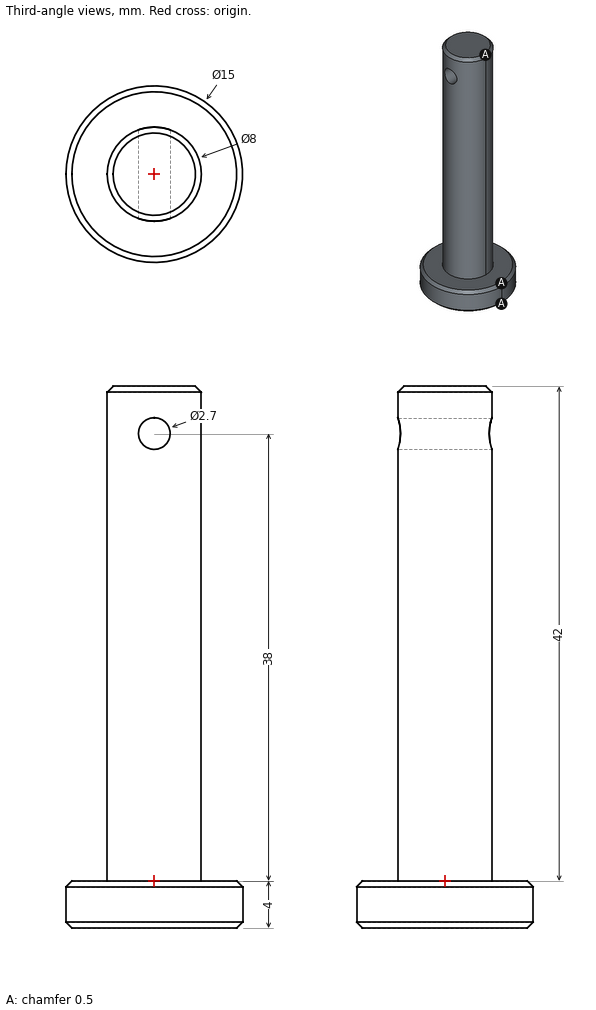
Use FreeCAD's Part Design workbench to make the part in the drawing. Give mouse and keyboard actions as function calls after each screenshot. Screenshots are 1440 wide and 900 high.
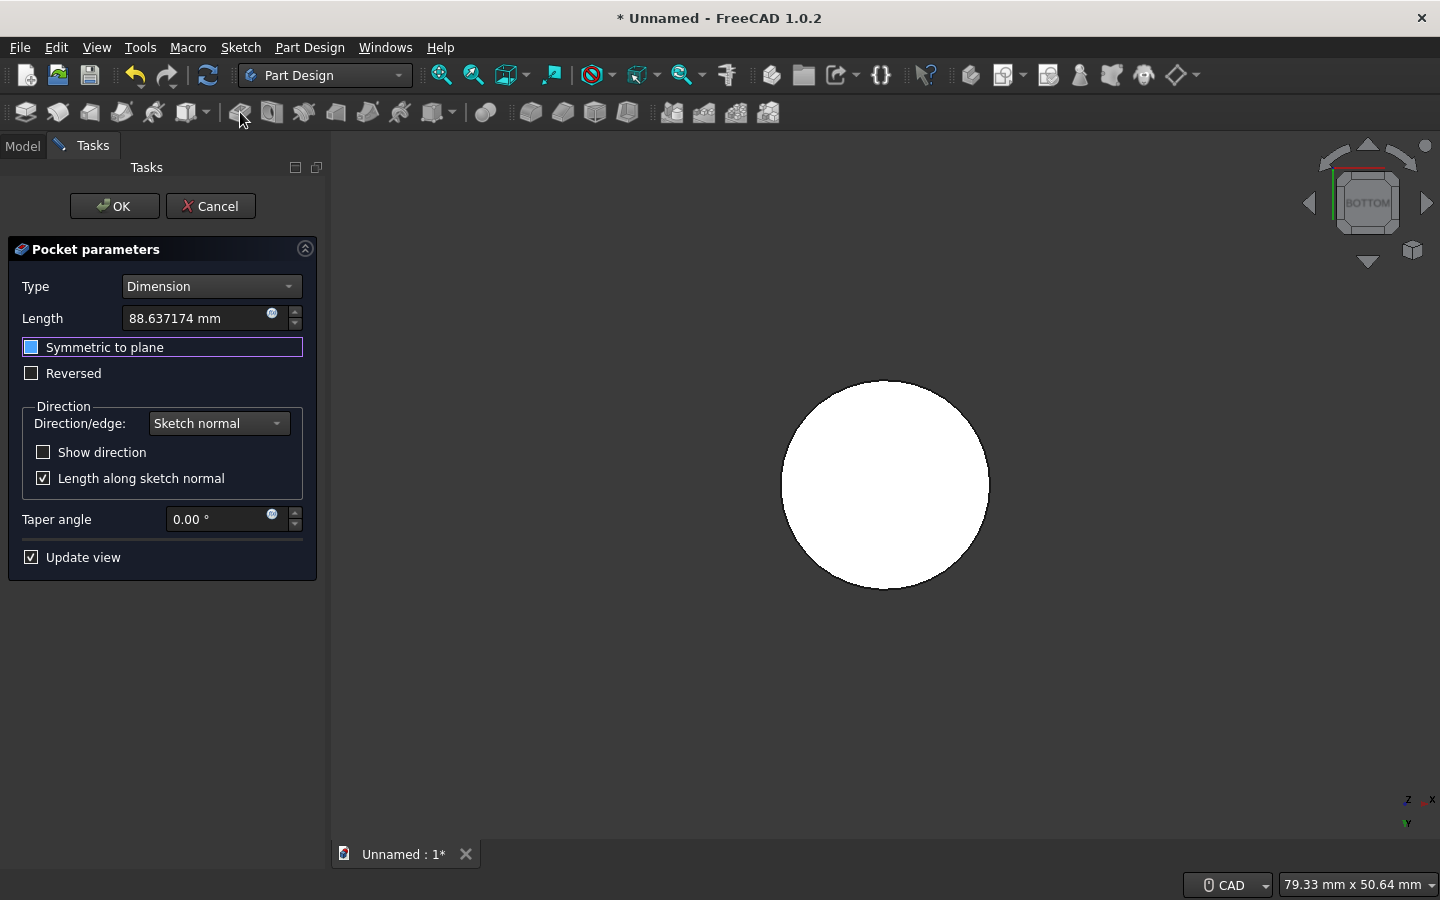
click(30, 347)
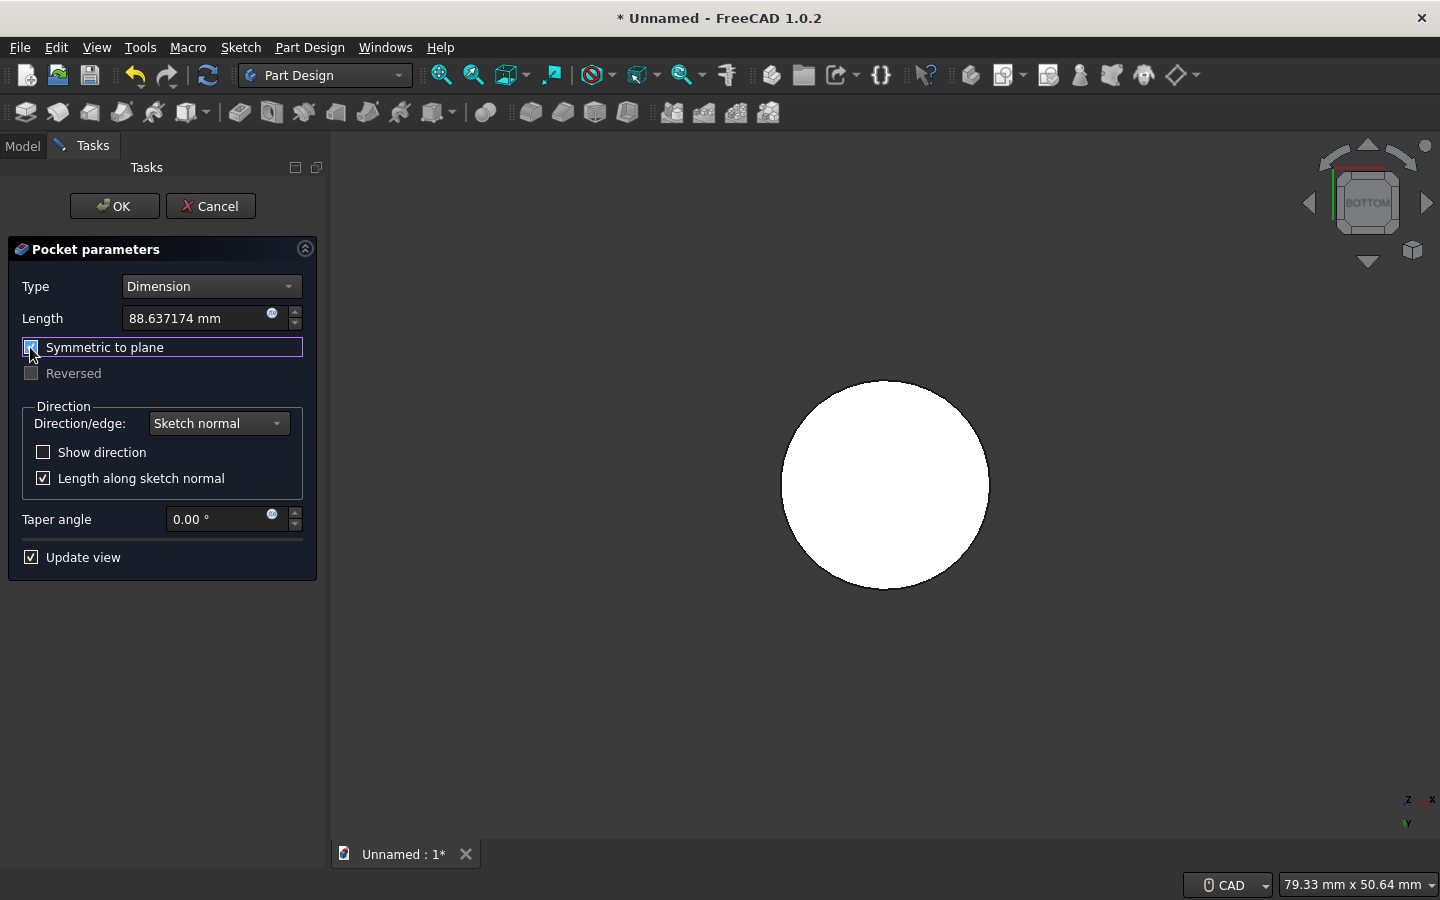
click(115, 206)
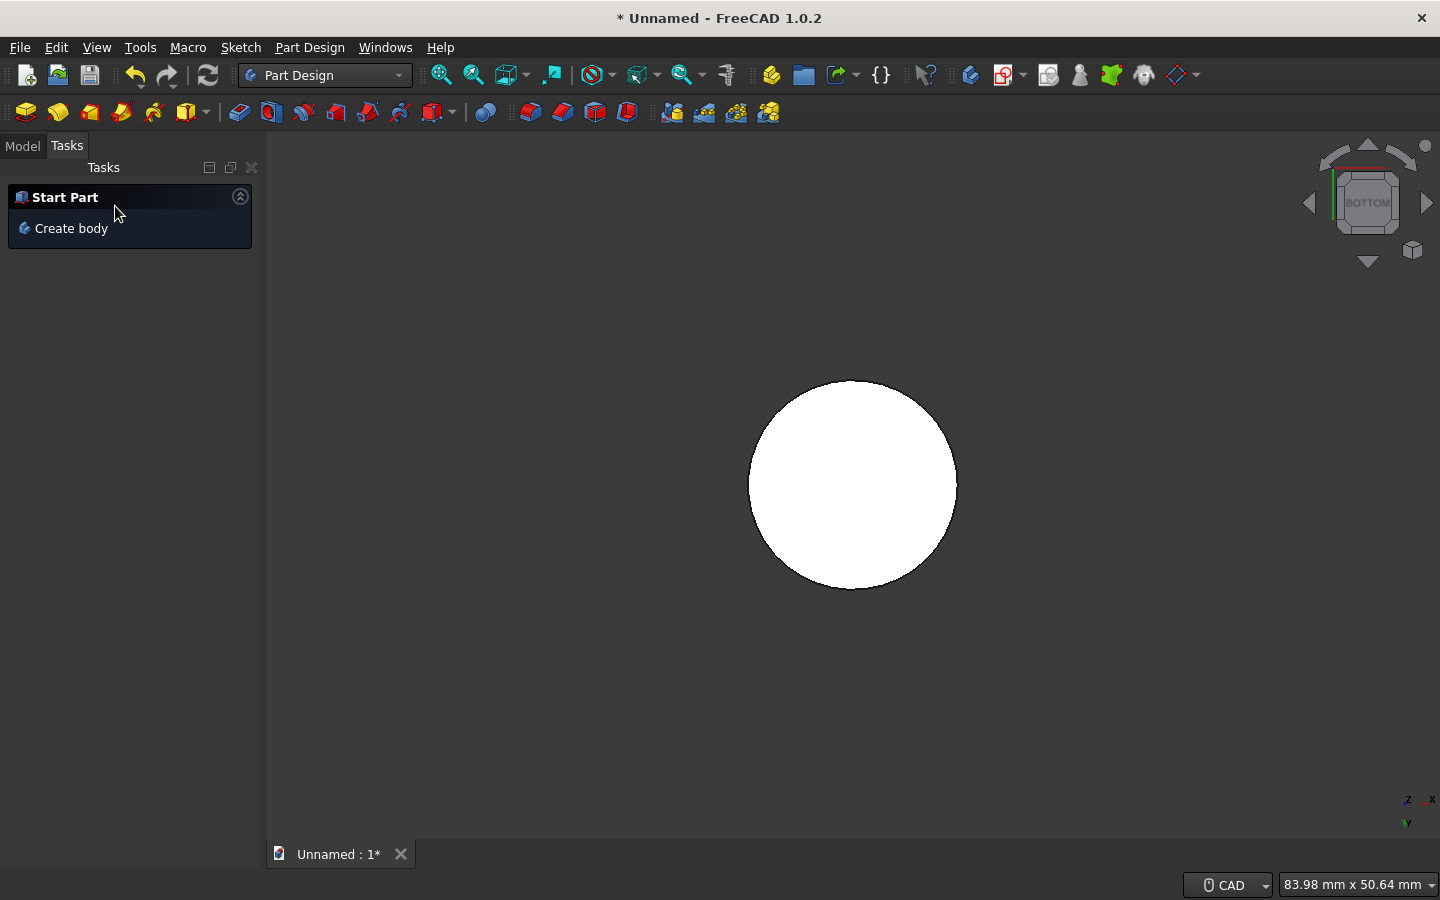
key(v)
key(f)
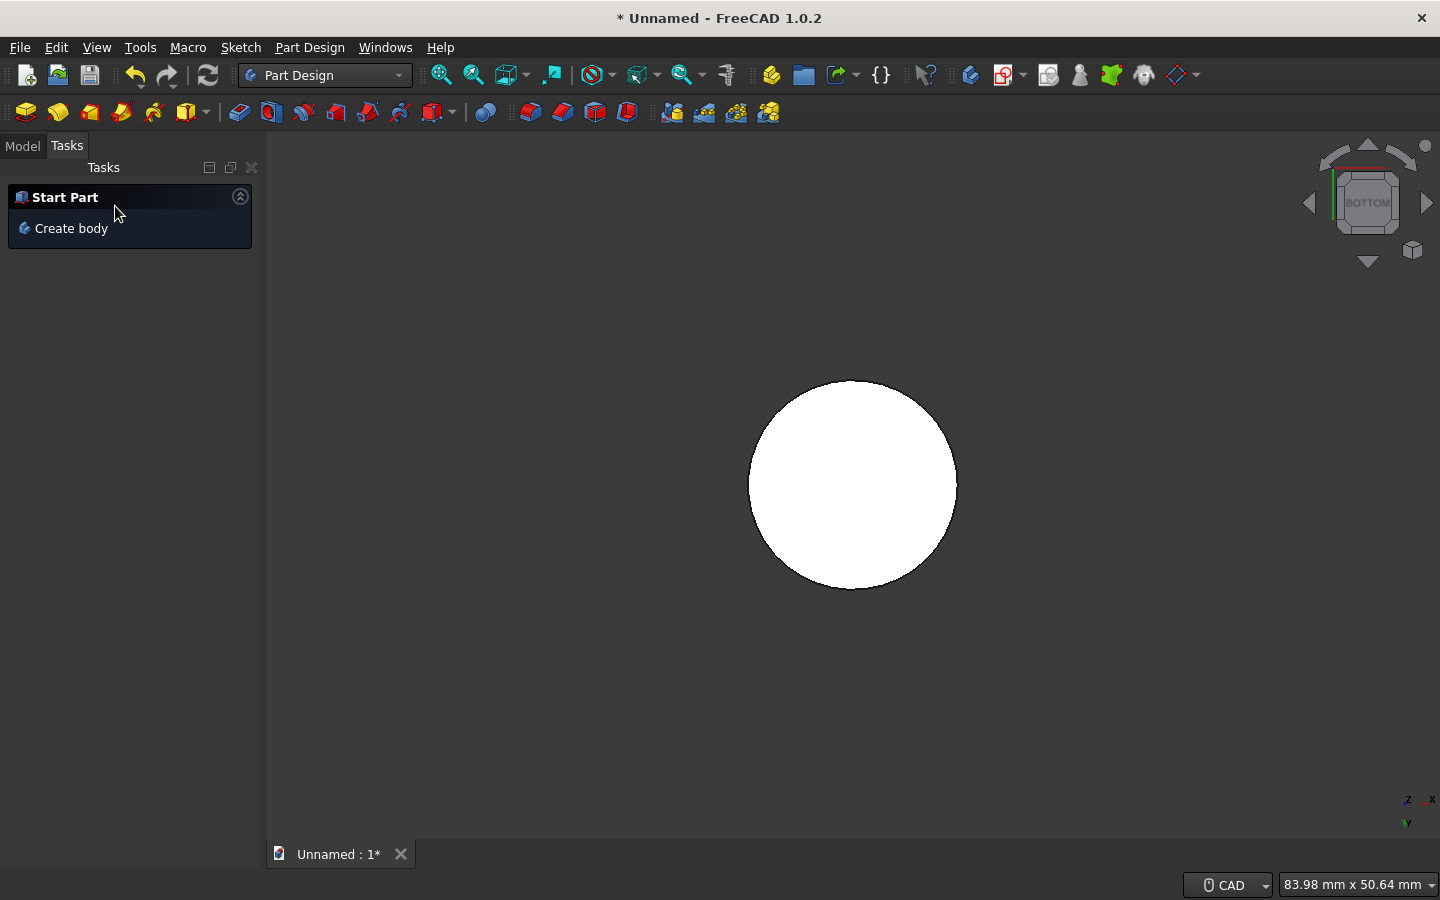
click(748, 484)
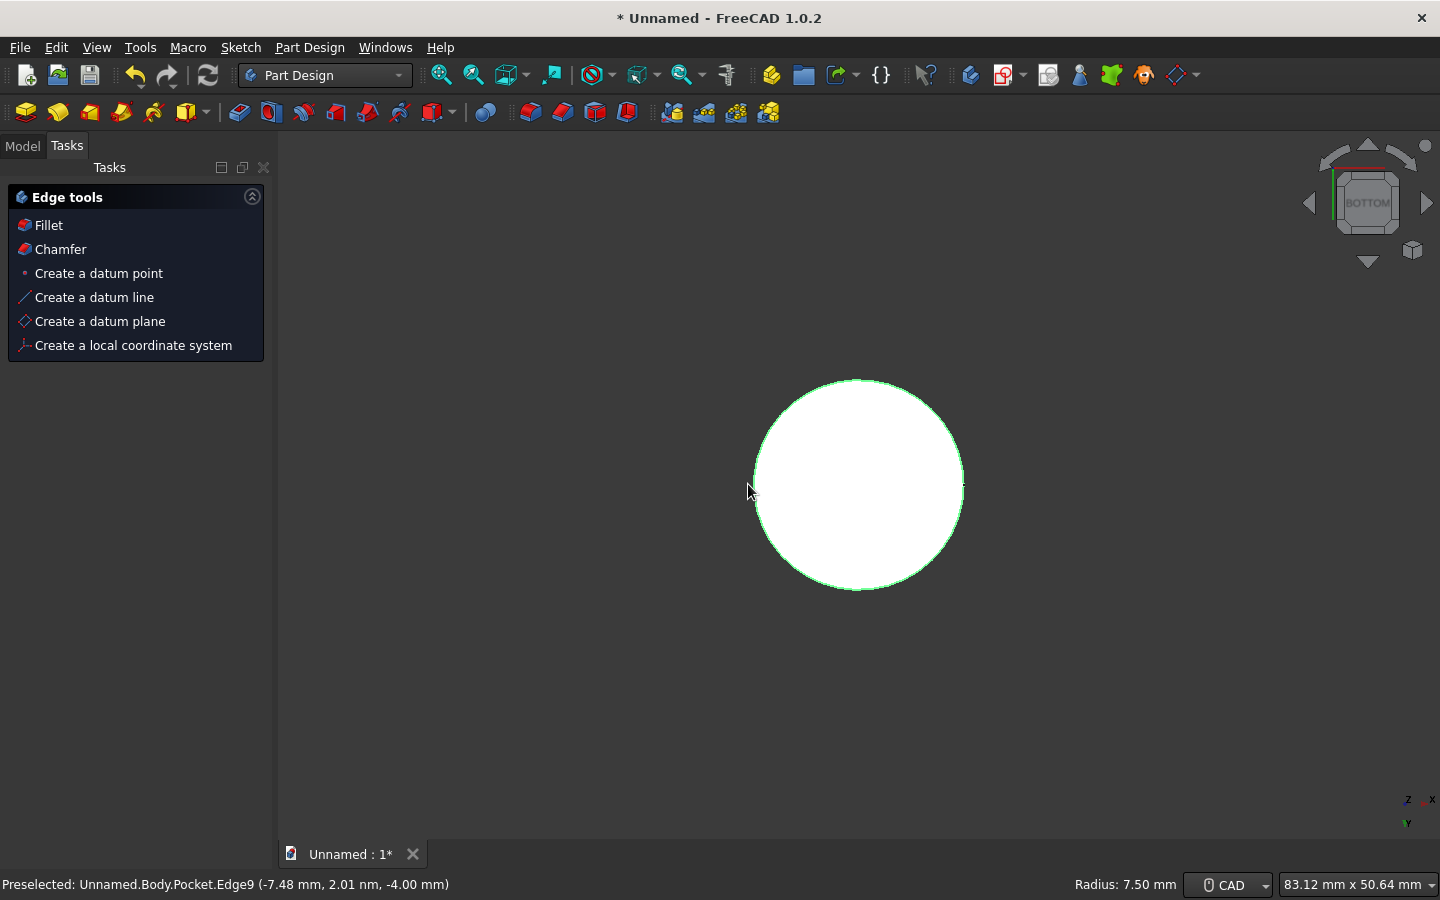
key(0)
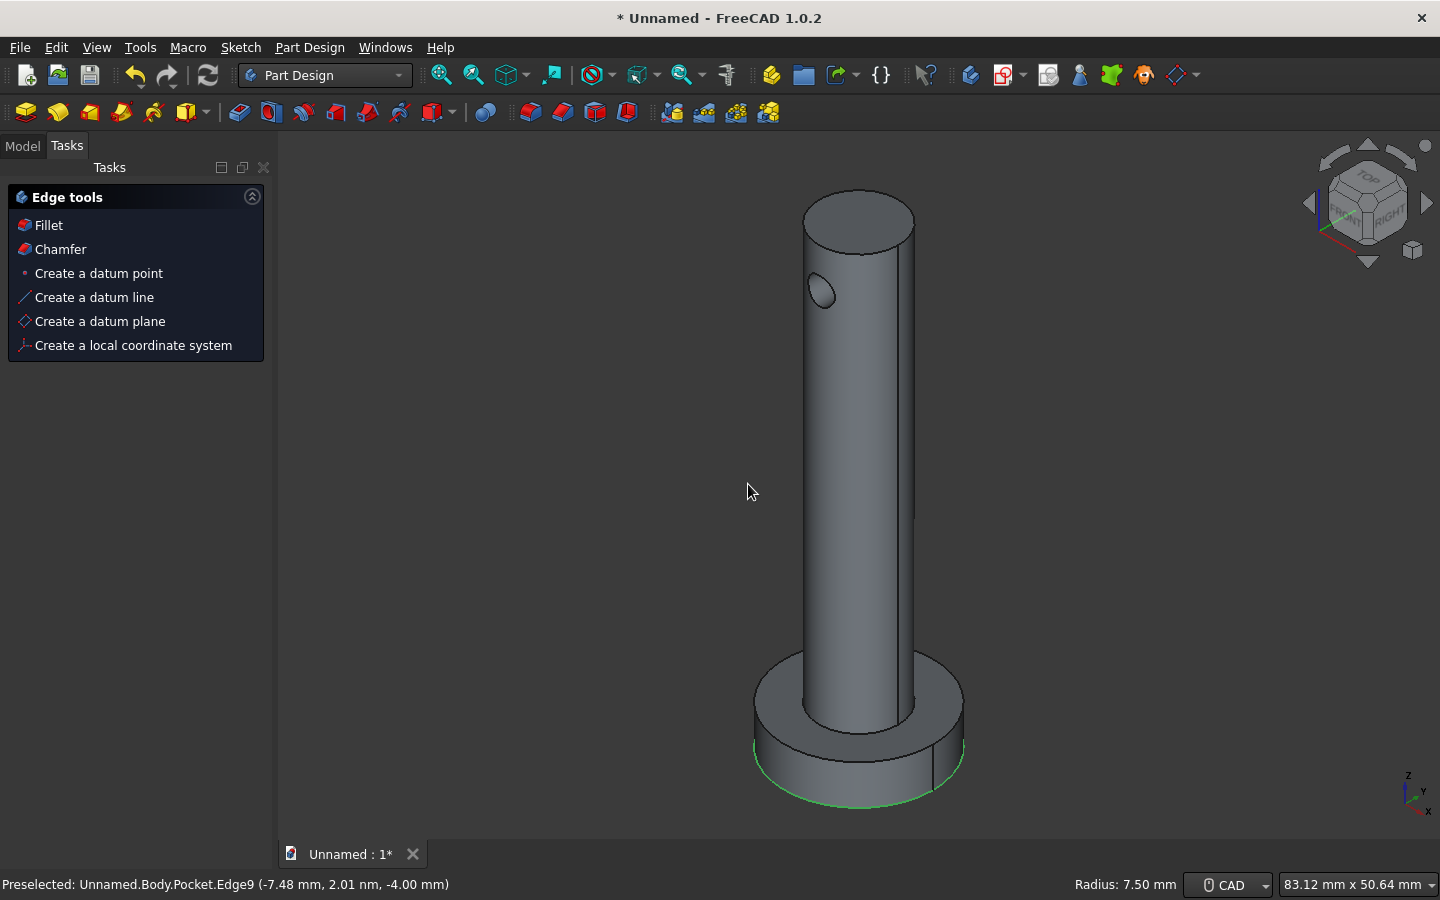
click(809, 236, ctrl)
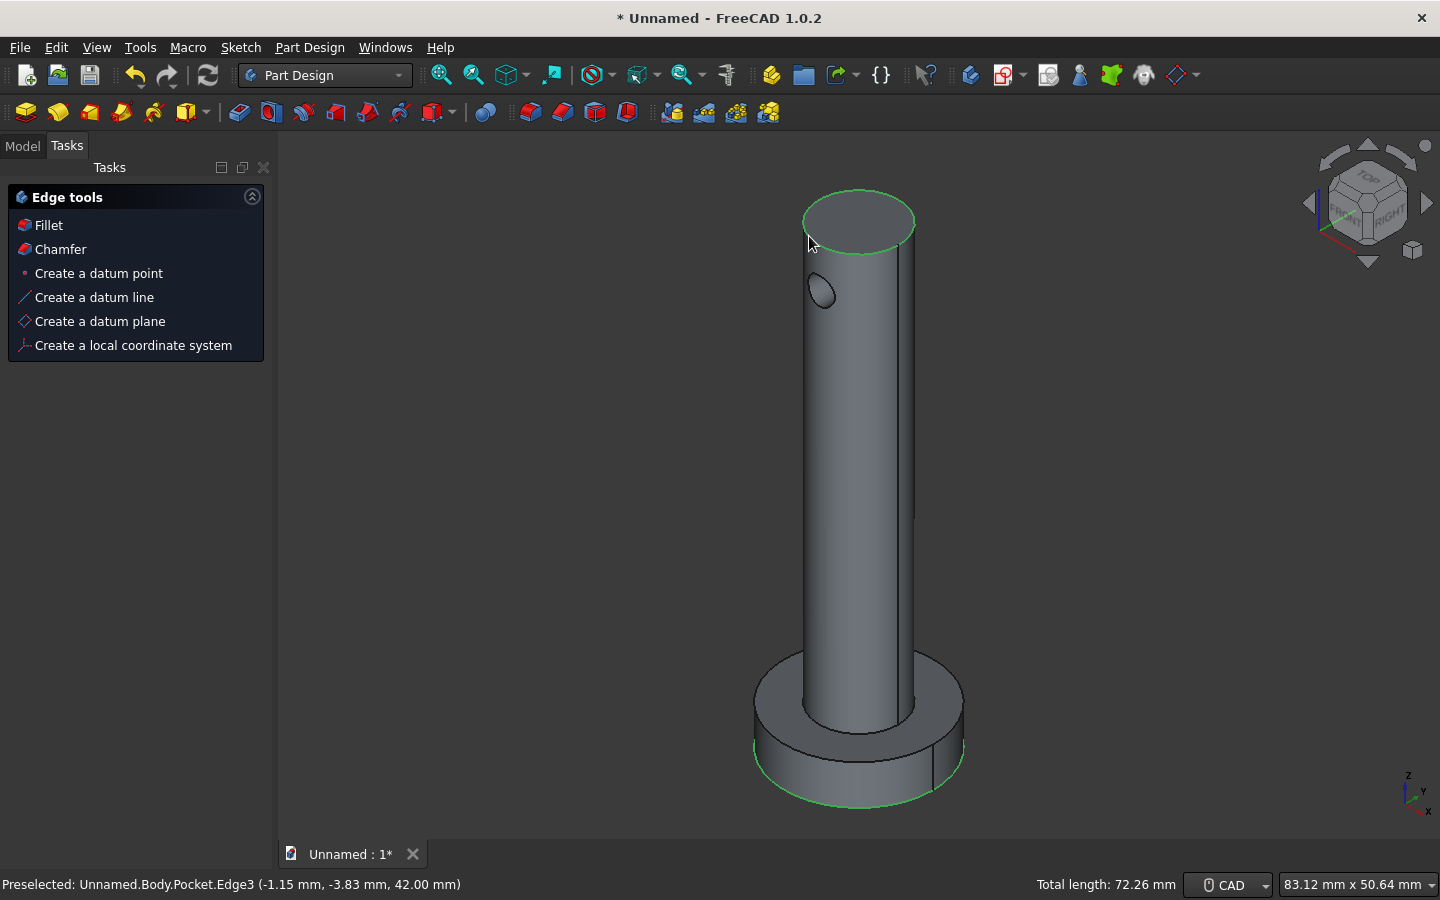
click(765, 728, ctrl)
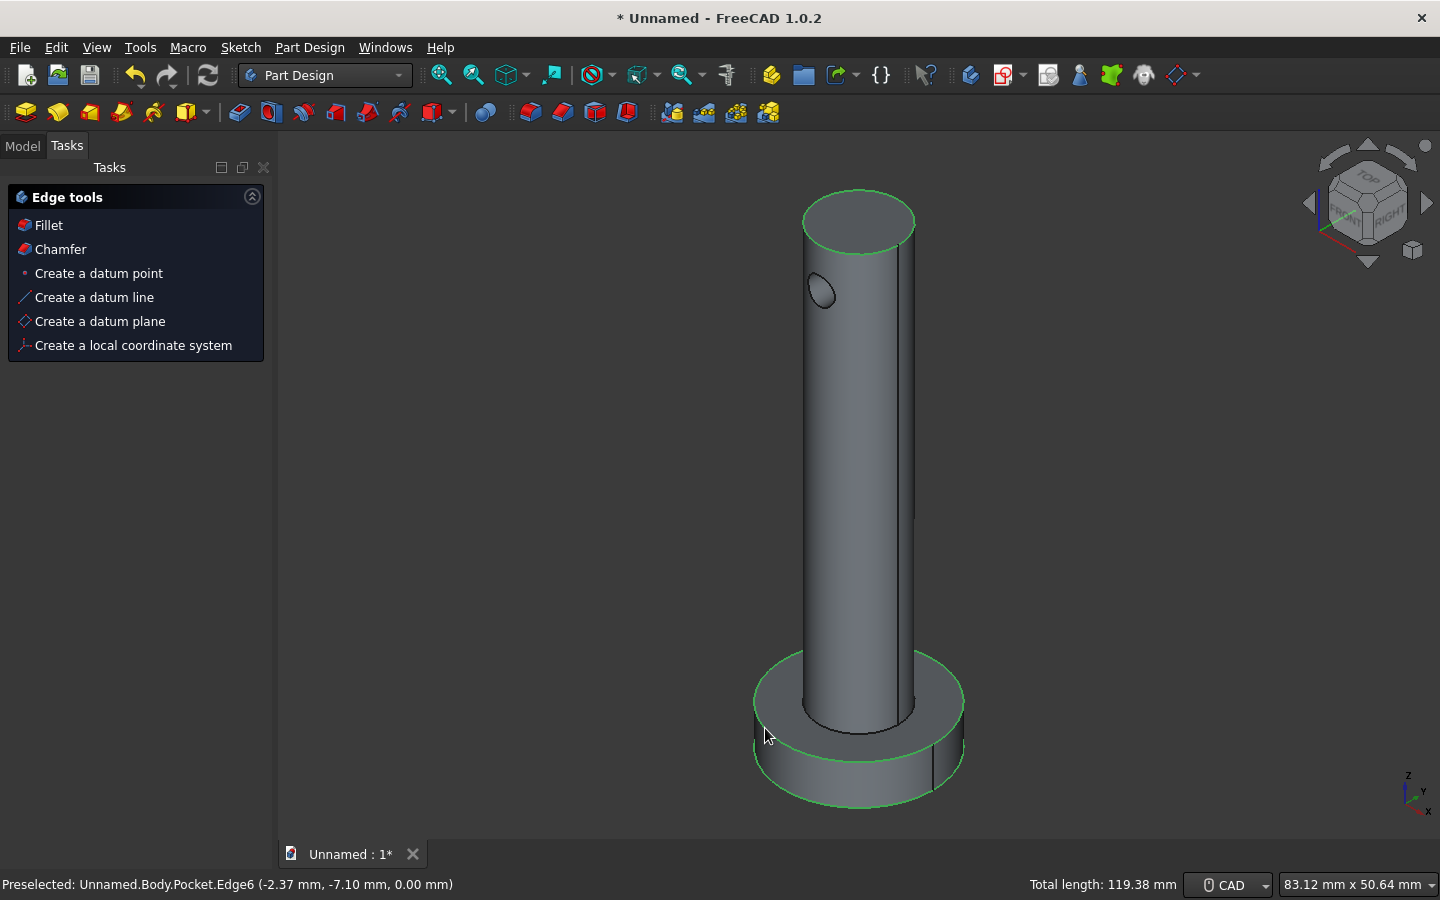
click(564, 112)